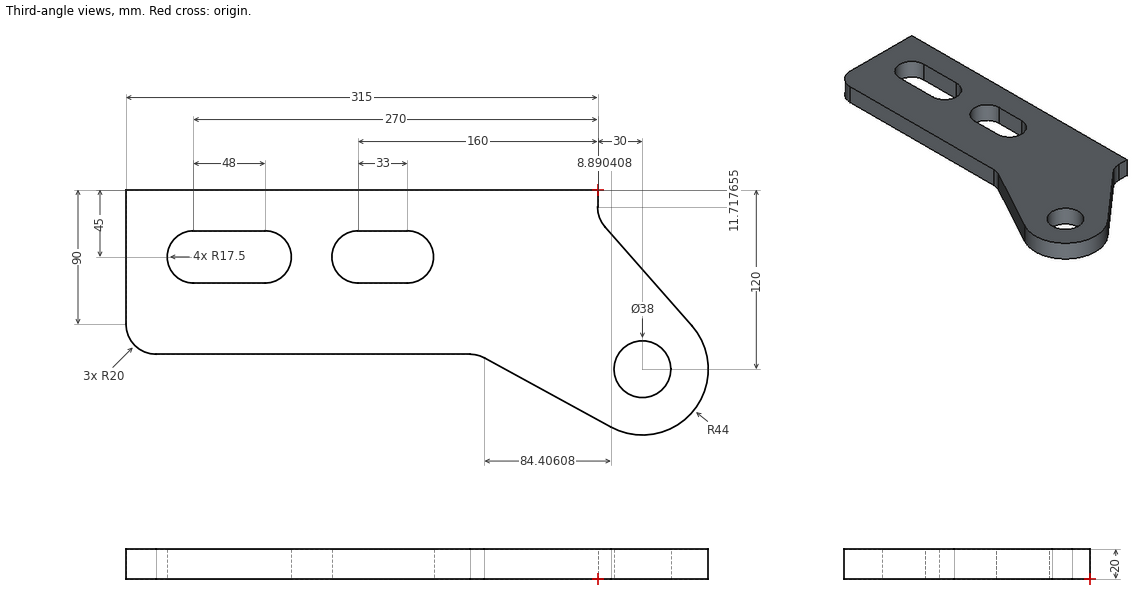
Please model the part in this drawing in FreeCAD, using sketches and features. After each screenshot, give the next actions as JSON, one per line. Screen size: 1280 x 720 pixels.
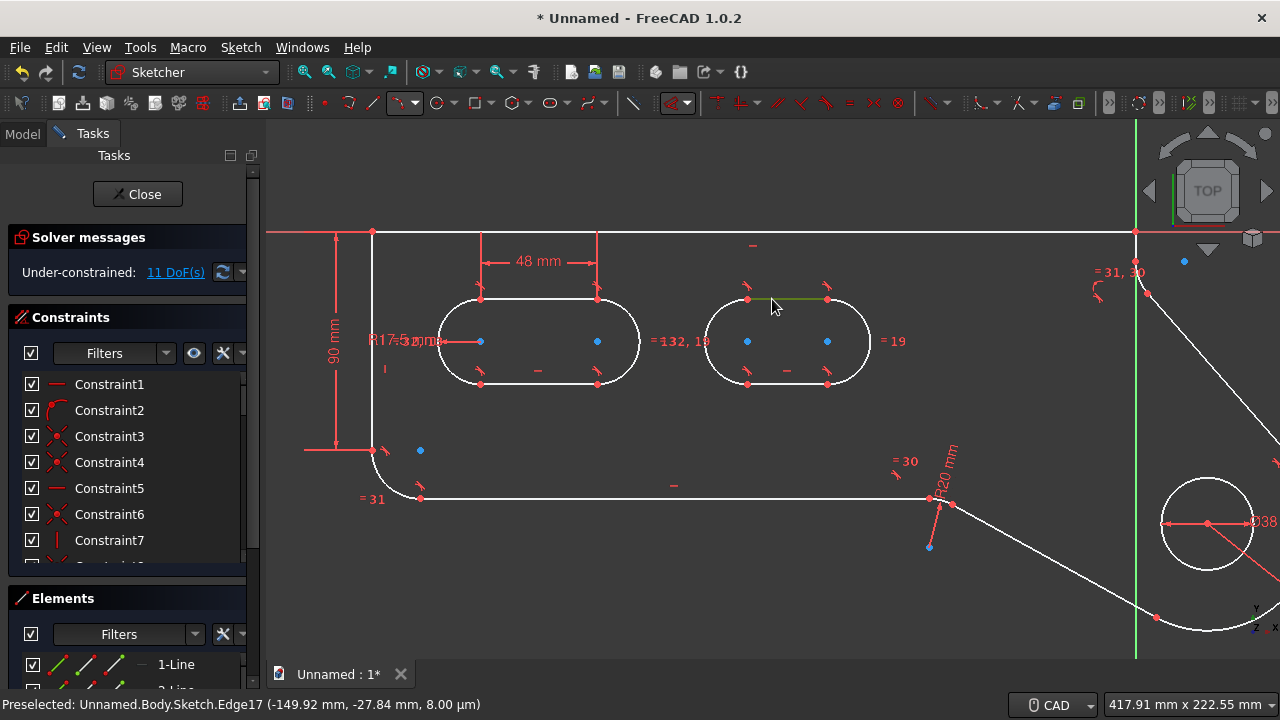
{"action": "key", "text": "l"}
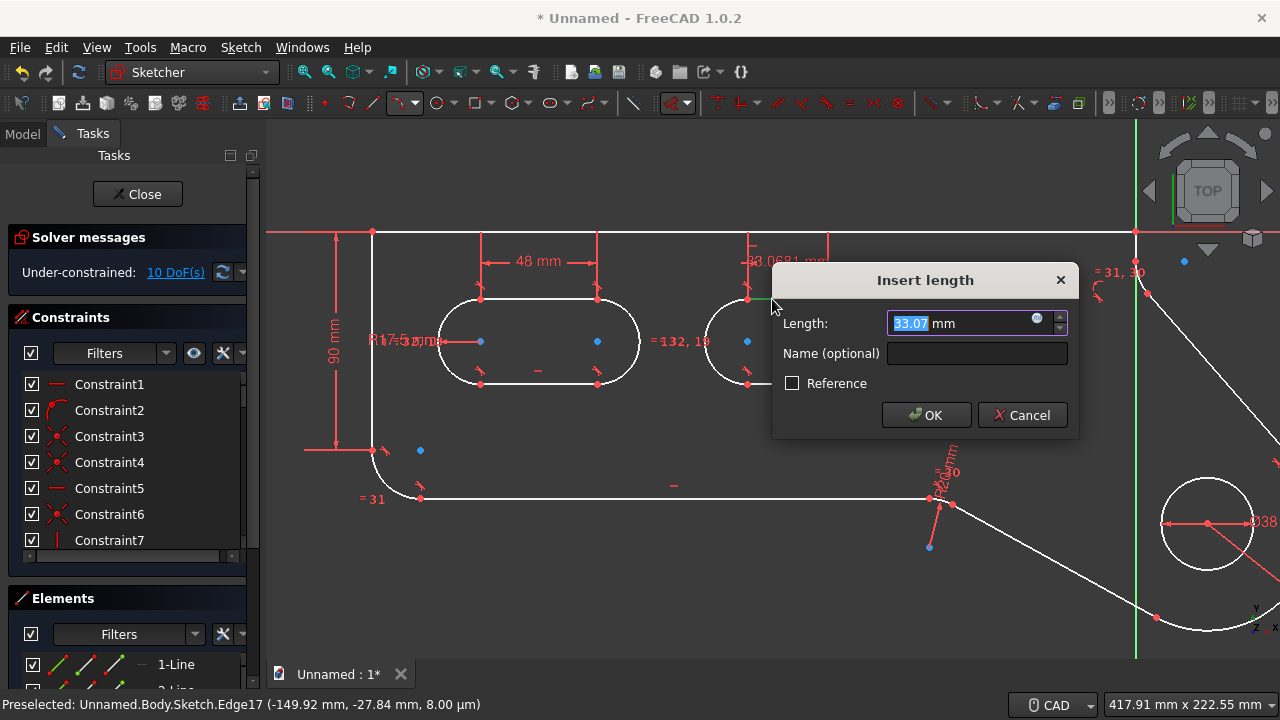
{"action": "type", "text": "33"}
{"action": "key", "text": "Return"}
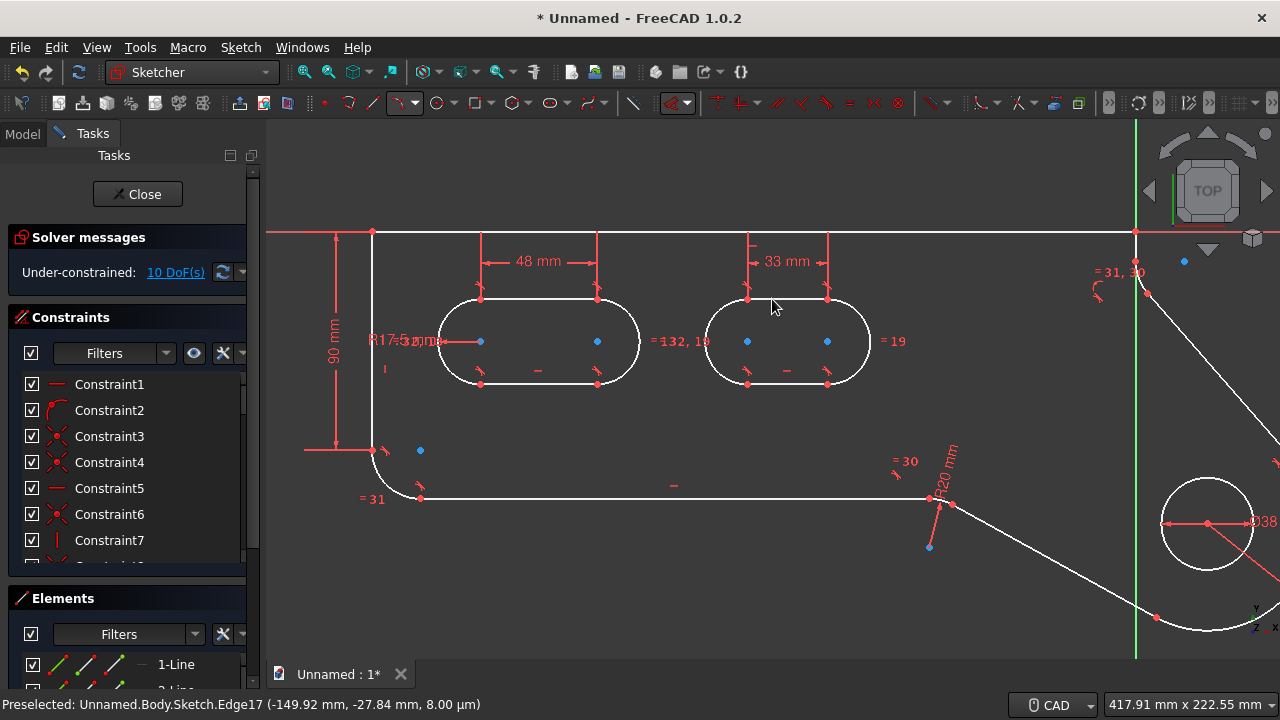
{"action": "scroll", "coordinate": [446, 317], "scroll_direction": "down", "scroll_amount": 2}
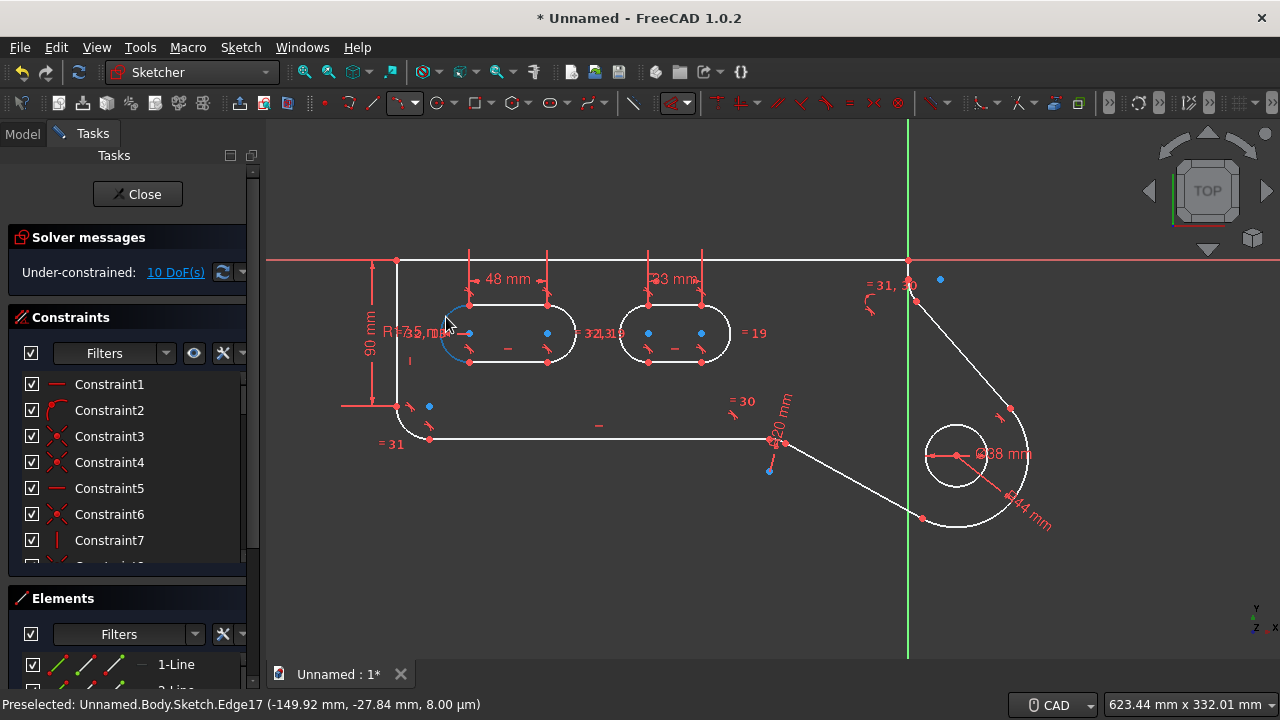
{"action": "left_click", "coordinate": [956, 456]}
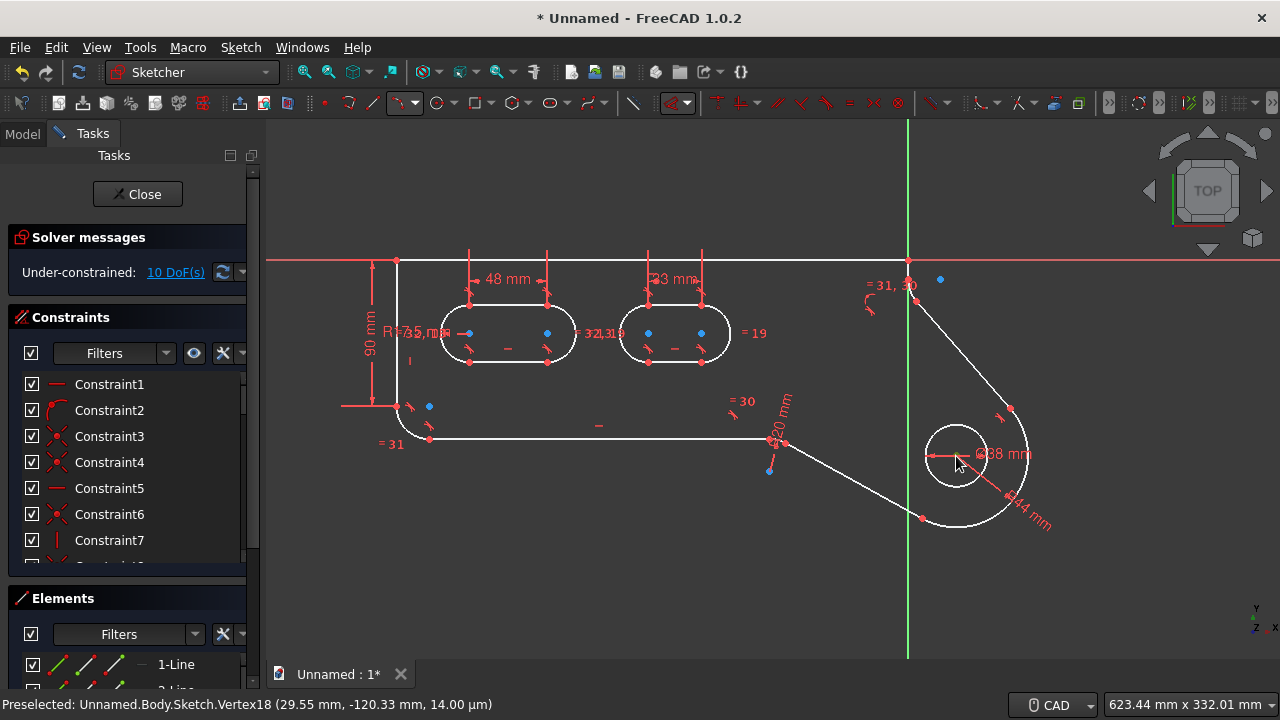
{"action": "left_click", "coordinate": [690, 104]}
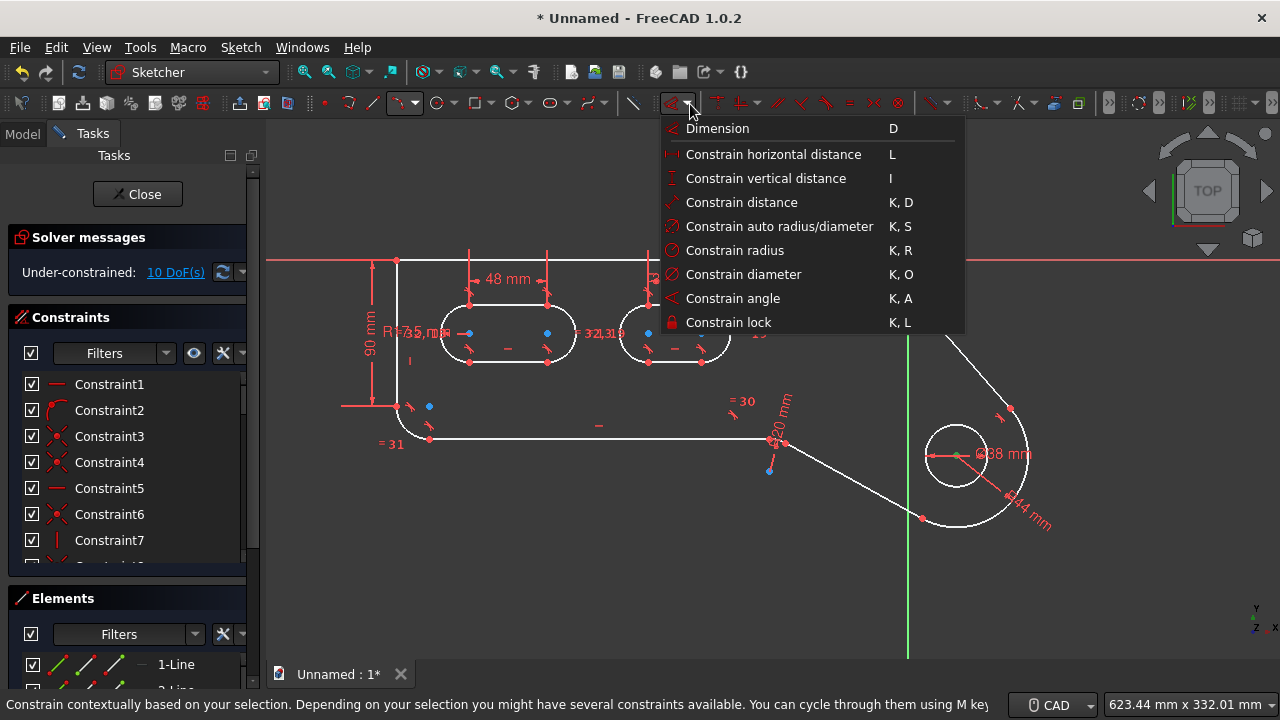
{"action": "left_click", "coordinate": [813, 154]}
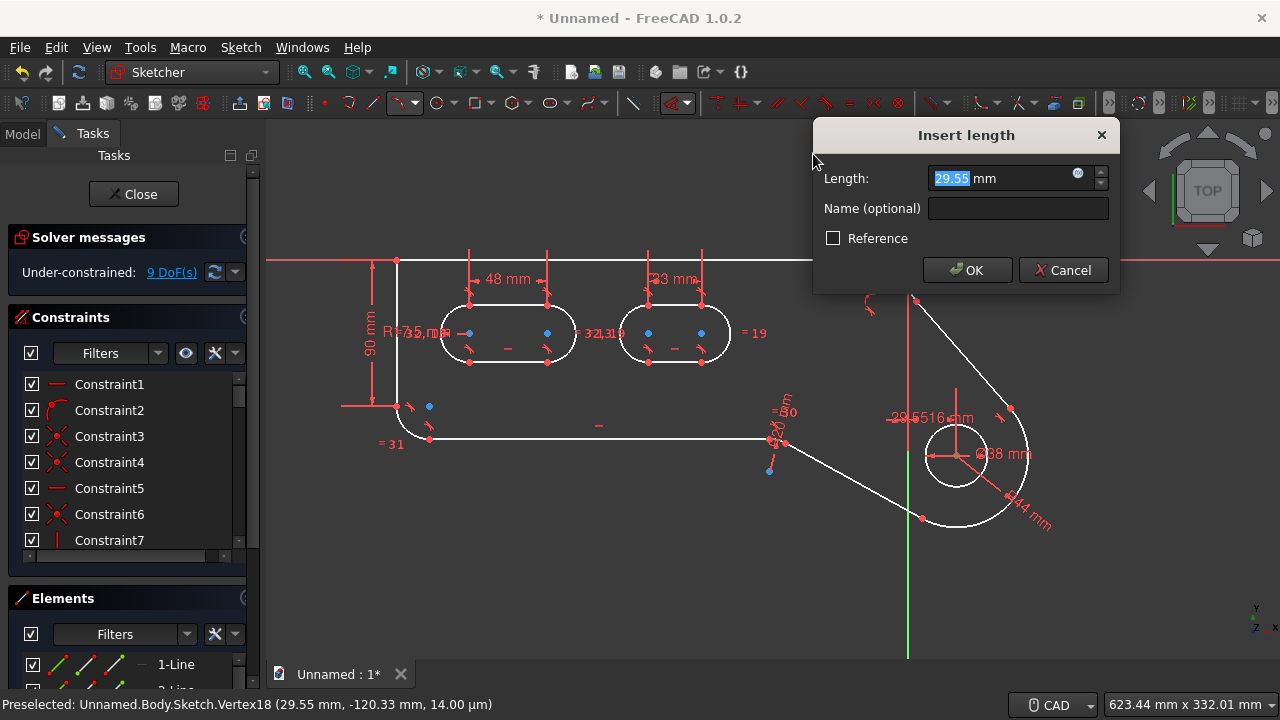
{"action": "type", "text": "30"}
{"action": "key", "text": "Return"}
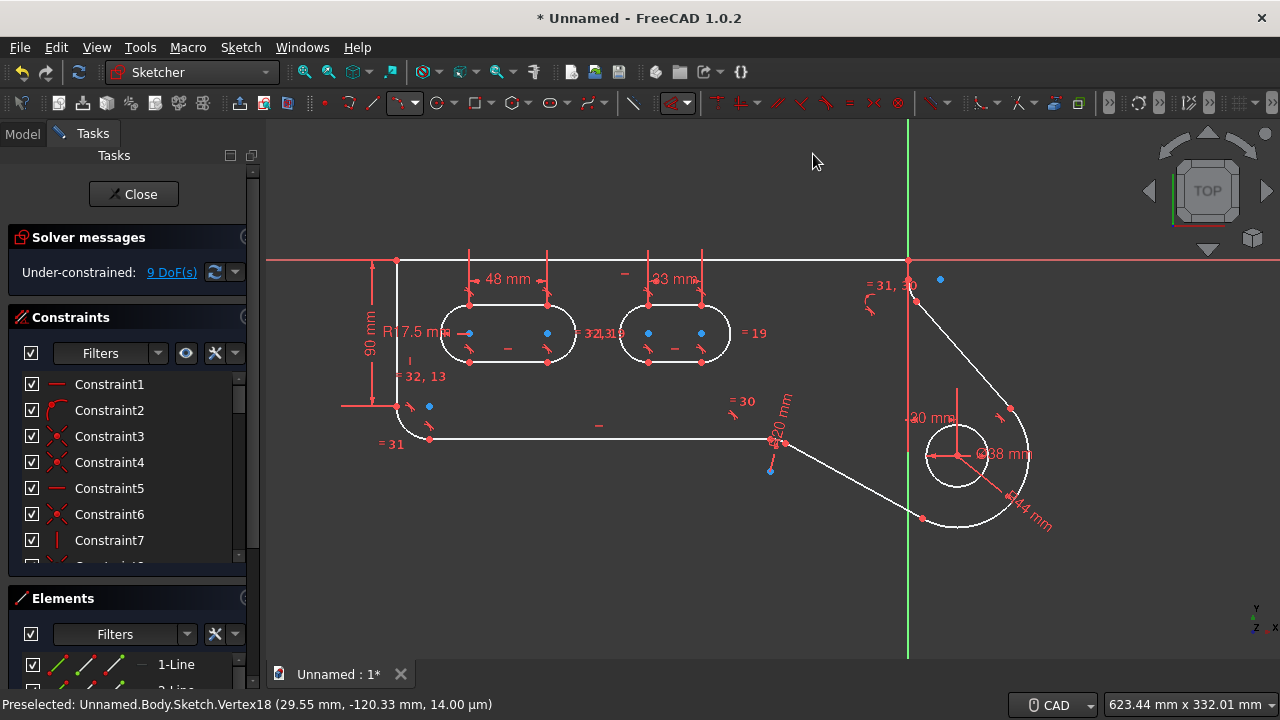
{"action": "left_click", "coordinate": [755, 260]}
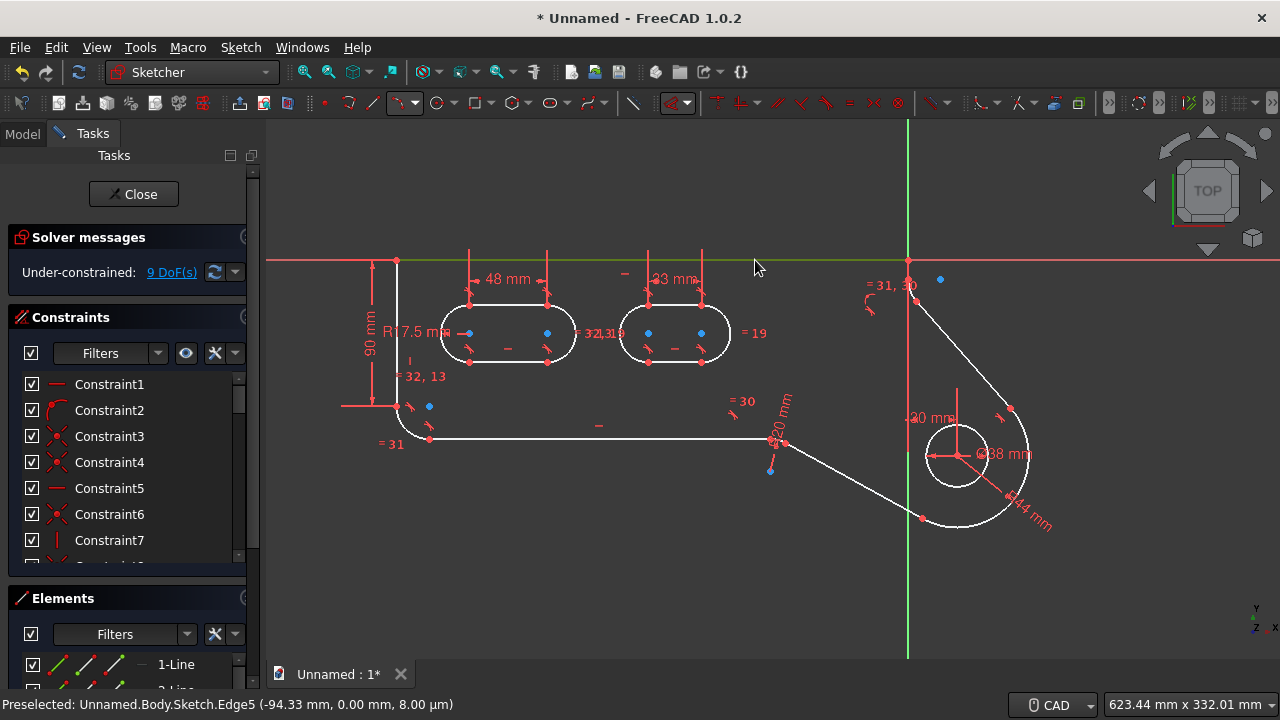
{"action": "key", "text": "l"}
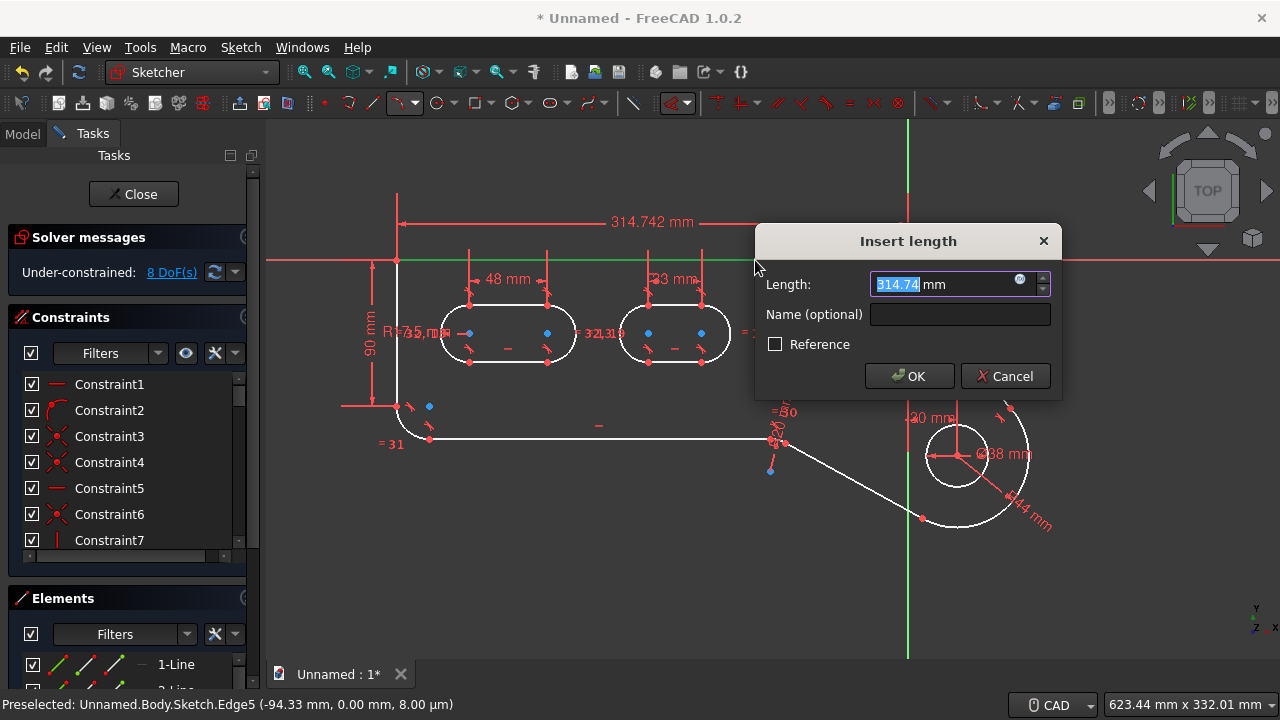
{"action": "type", "text": "315"}
{"action": "key", "text": "Return"}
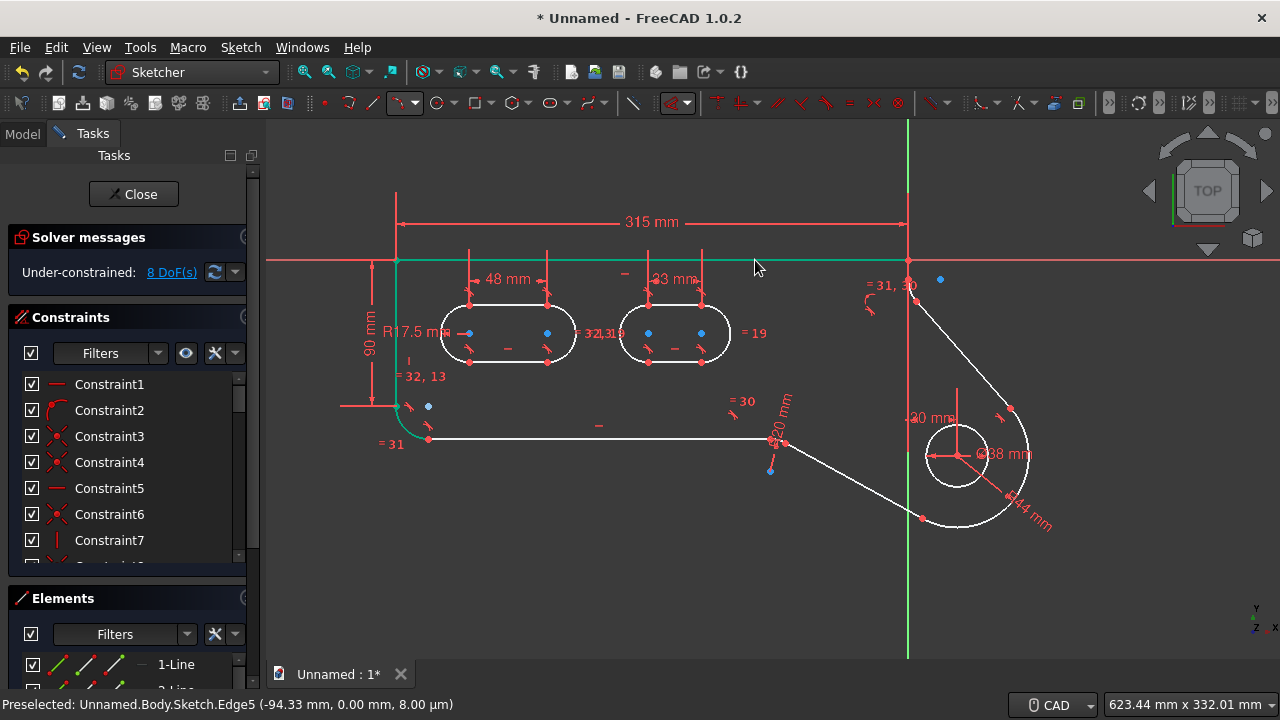
{"action": "left_click", "coordinate": [469, 334]}